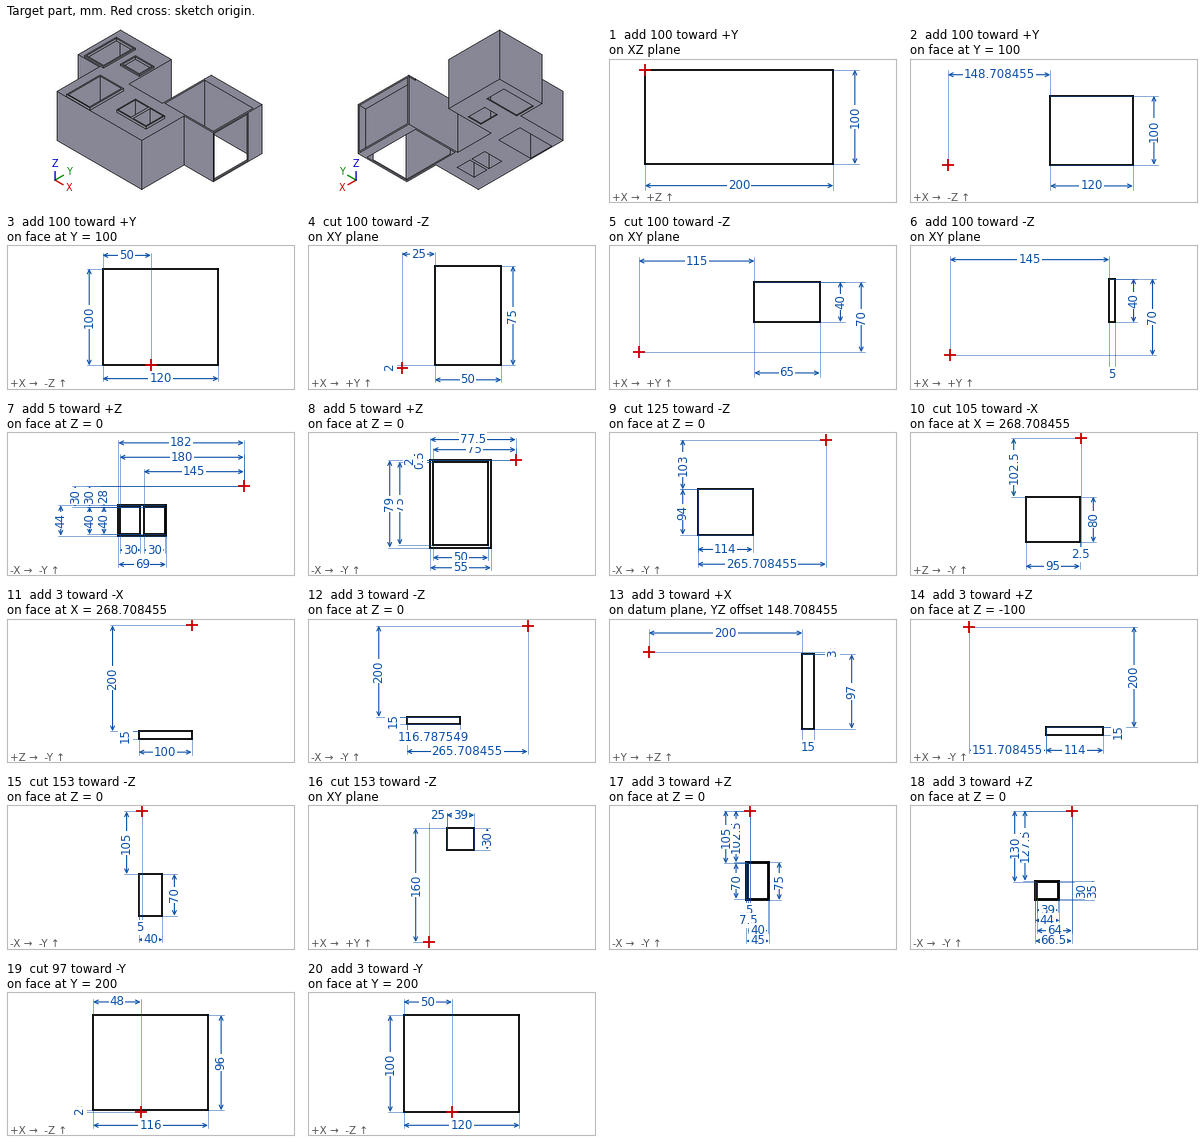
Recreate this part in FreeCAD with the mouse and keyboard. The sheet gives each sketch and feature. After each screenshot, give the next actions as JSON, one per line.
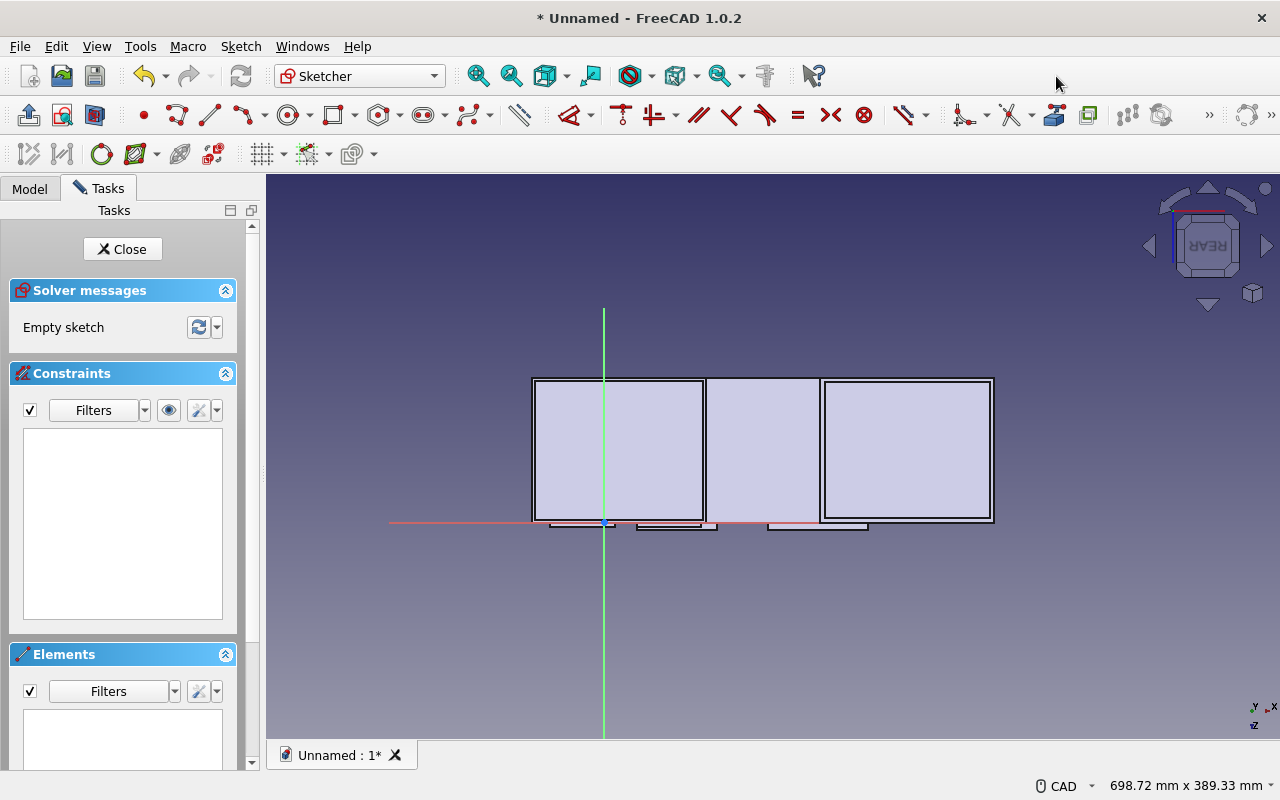
{"action": "scroll", "coordinate": [569, 447], "scroll_direction": "up", "scroll_amount": 5}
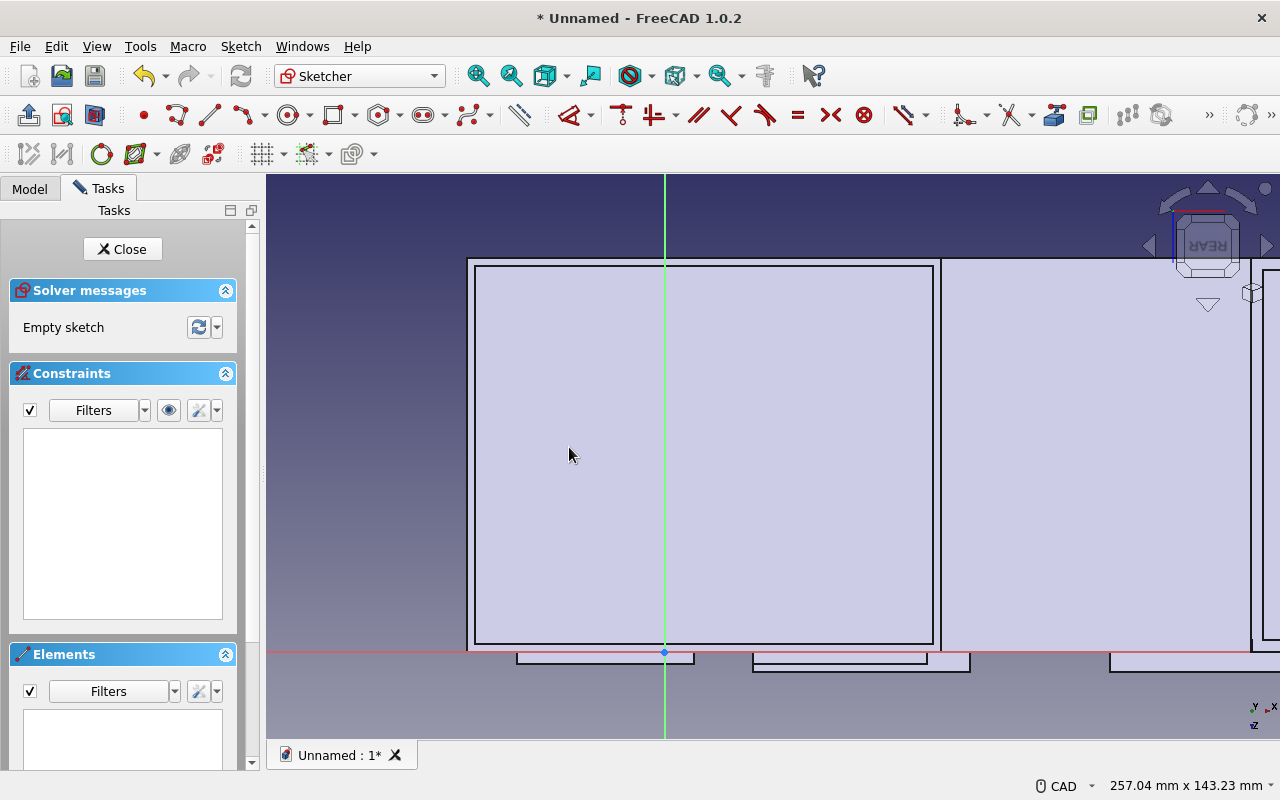
{"action": "left_click", "coordinate": [332, 116]}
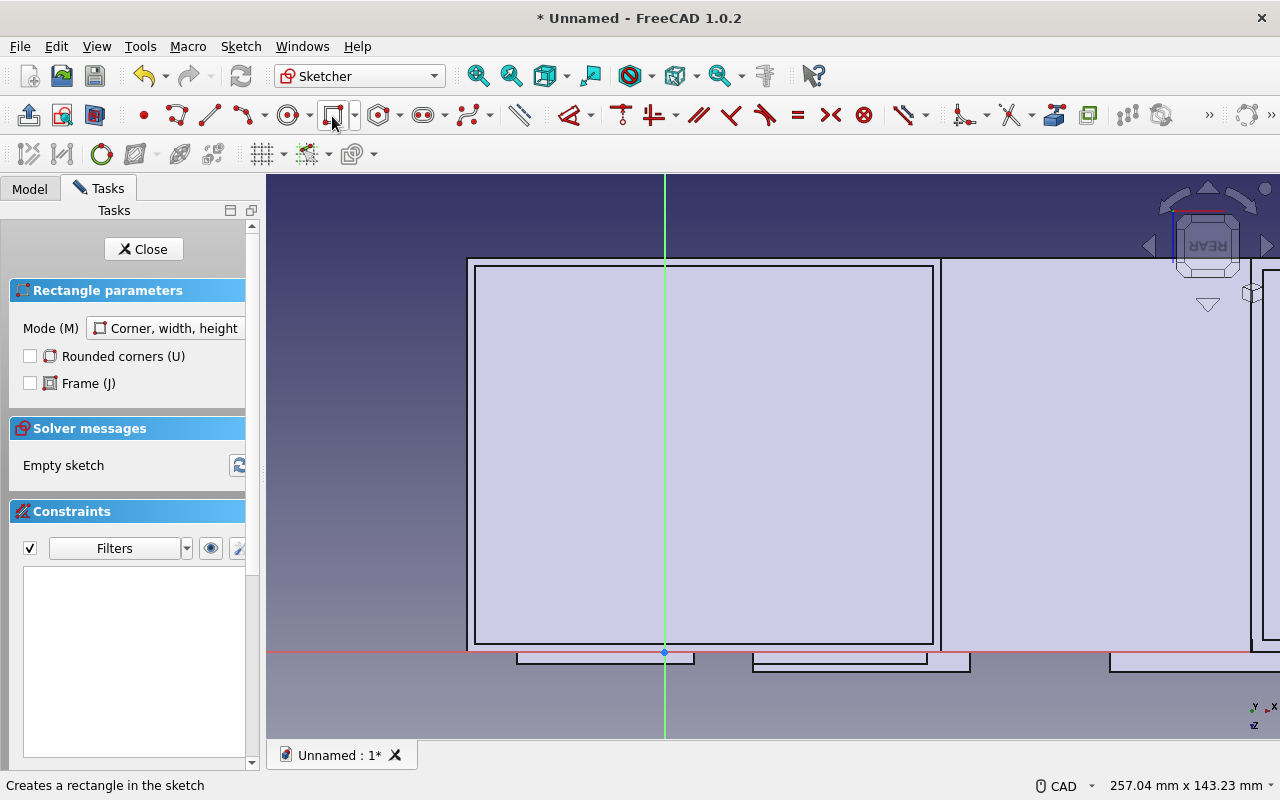
{"action": "left_click", "coordinate": [467, 258]}
{"action": "left_click", "coordinate": [941, 652]}
{"action": "key", "text": "Escape"}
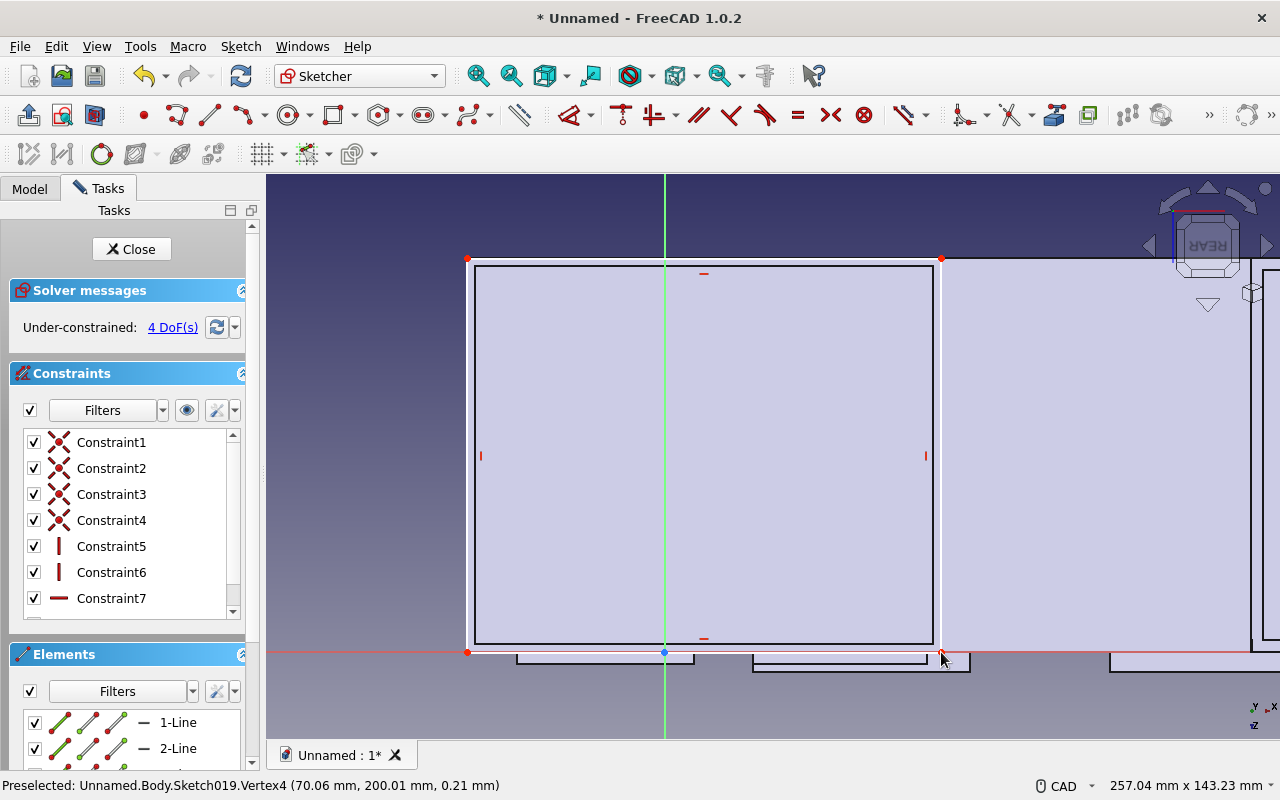
{"action": "left_click", "coordinate": [467, 653]}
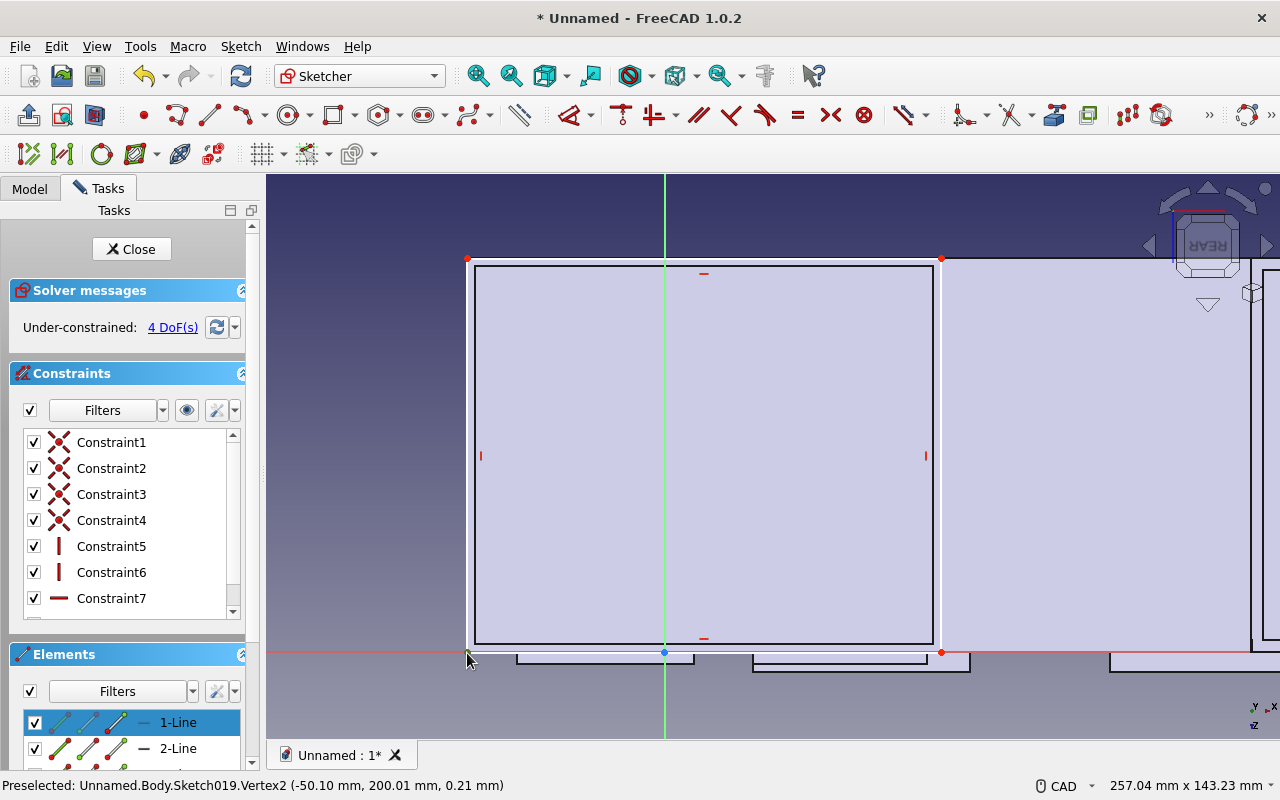
{"action": "left_click", "coordinate": [353, 652]}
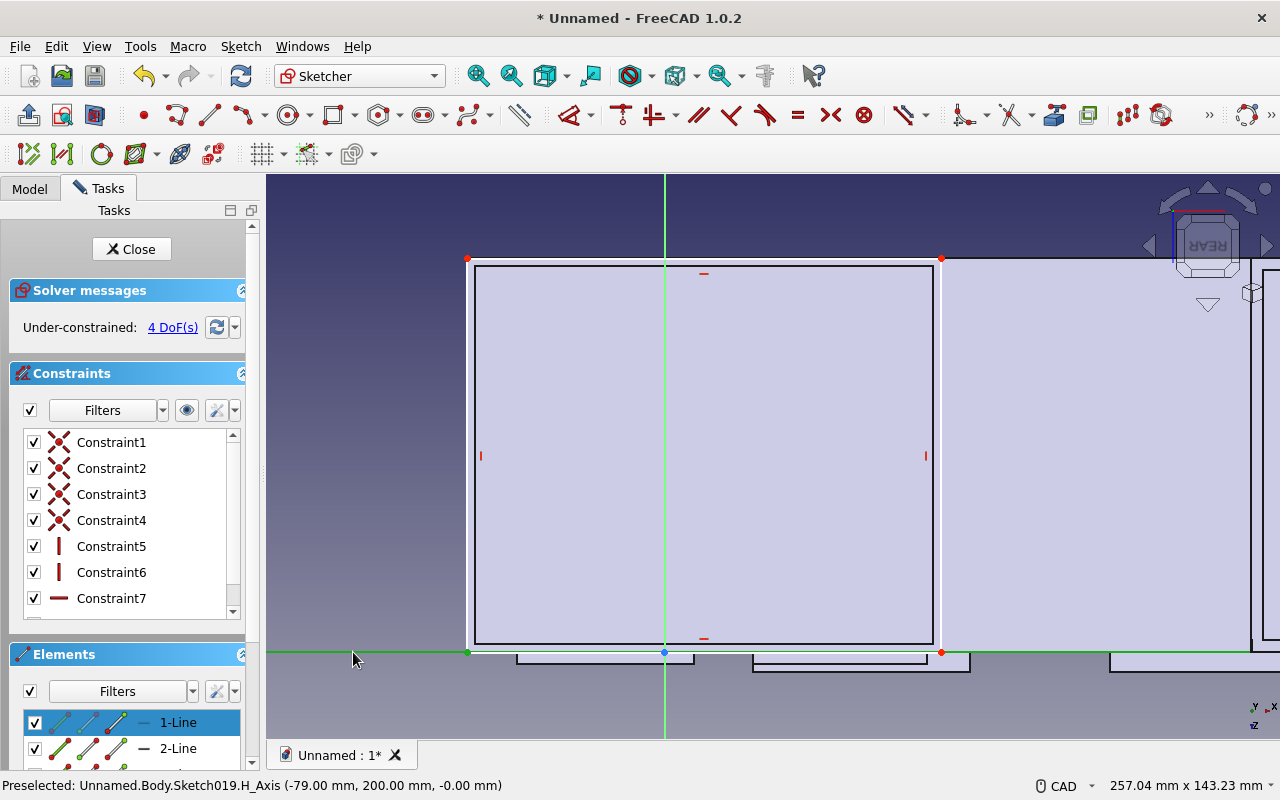
{"action": "left_click", "coordinate": [621, 116]}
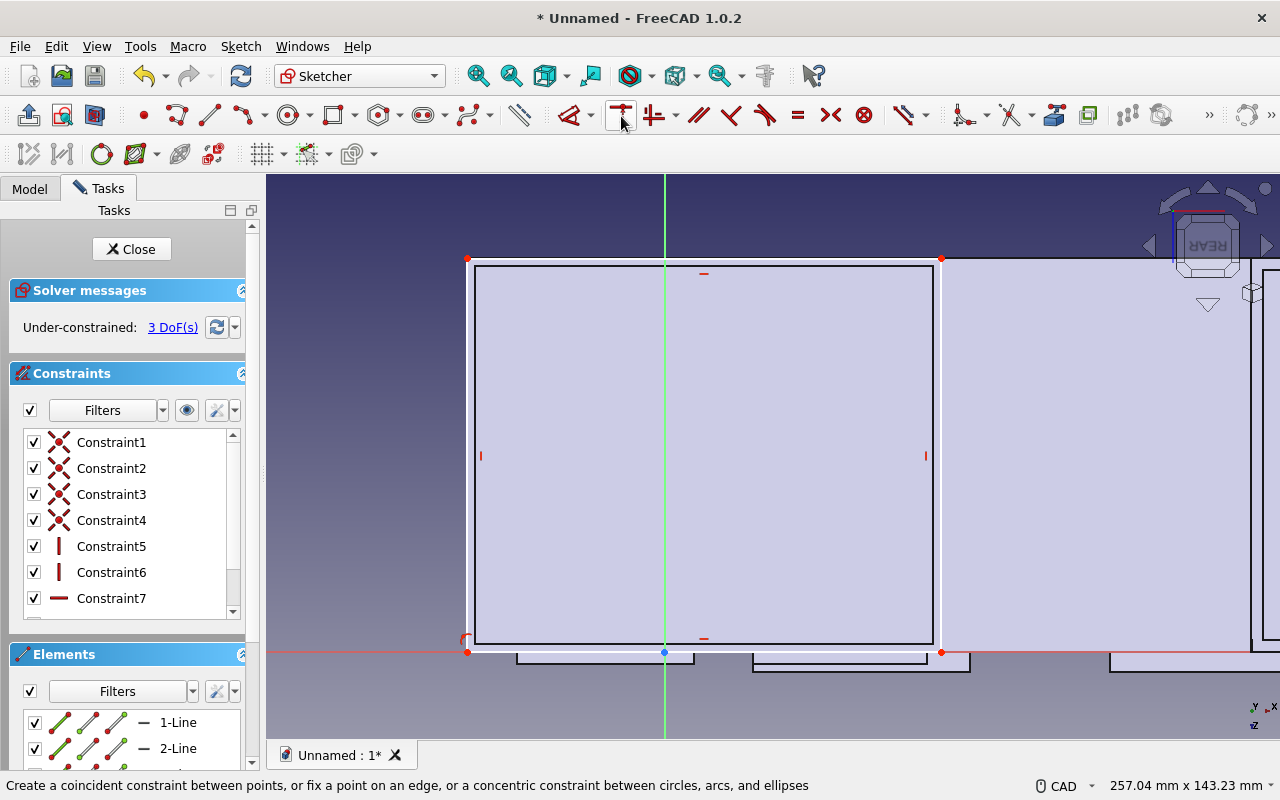
{"action": "left_click", "coordinate": [568, 116]}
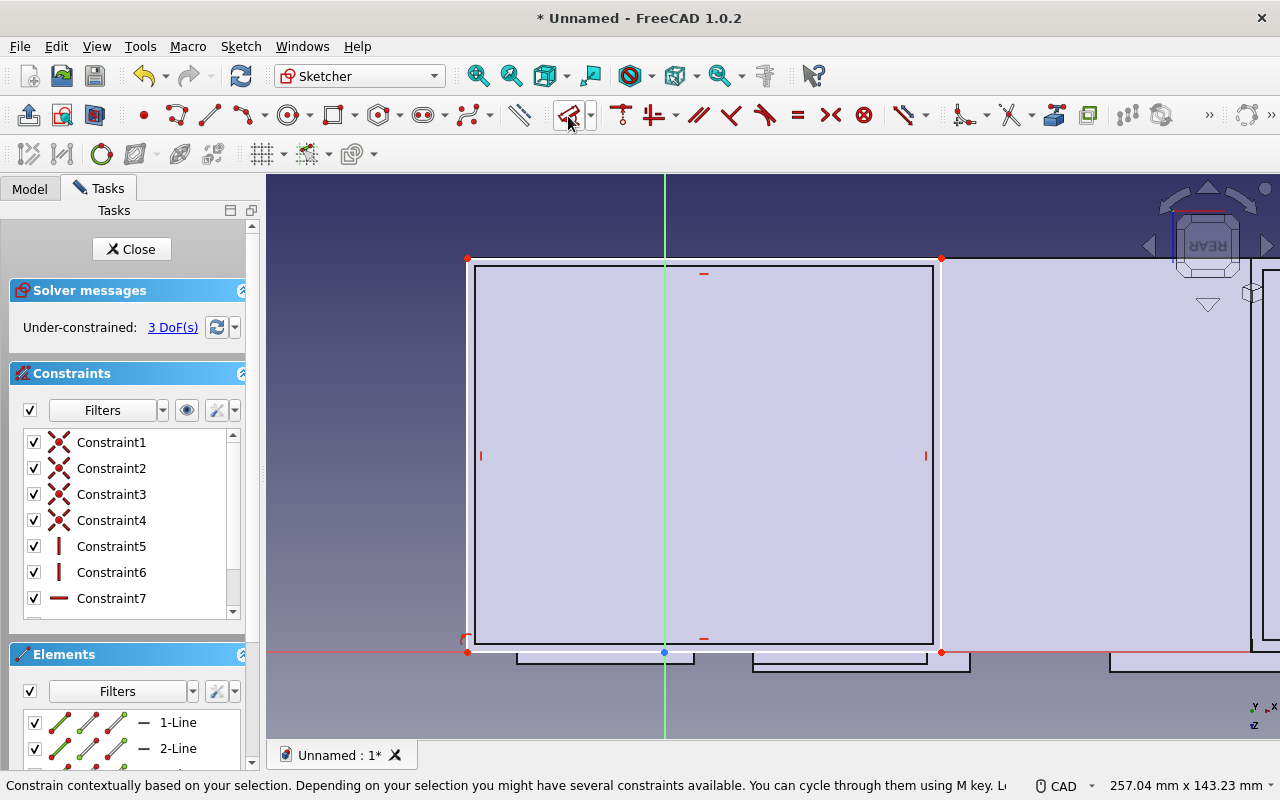
{"action": "left_click", "coordinate": [467, 377]}
{"action": "left_click", "coordinate": [433, 456]}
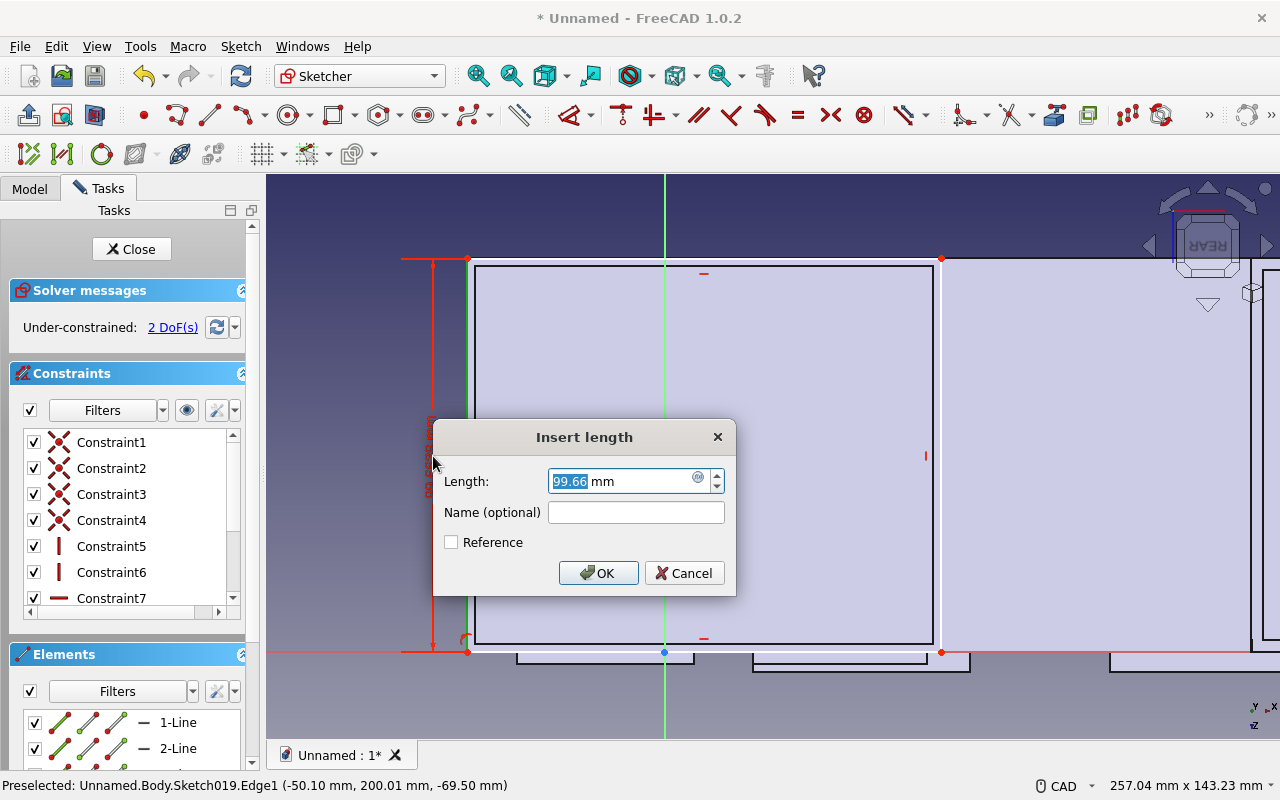
{"action": "type", "text": "100"}
{"action": "key", "text": "Return"}